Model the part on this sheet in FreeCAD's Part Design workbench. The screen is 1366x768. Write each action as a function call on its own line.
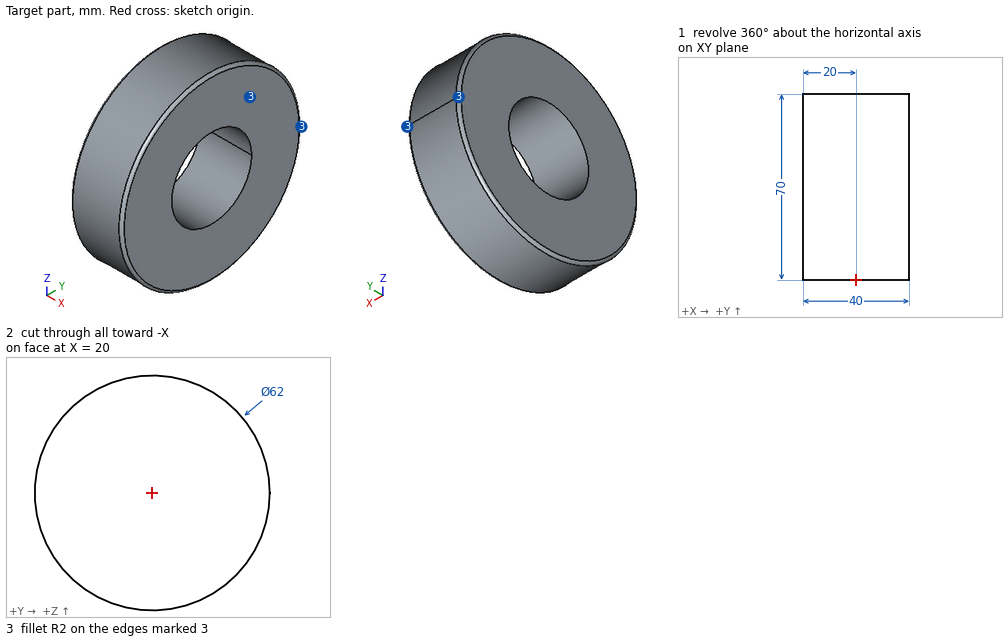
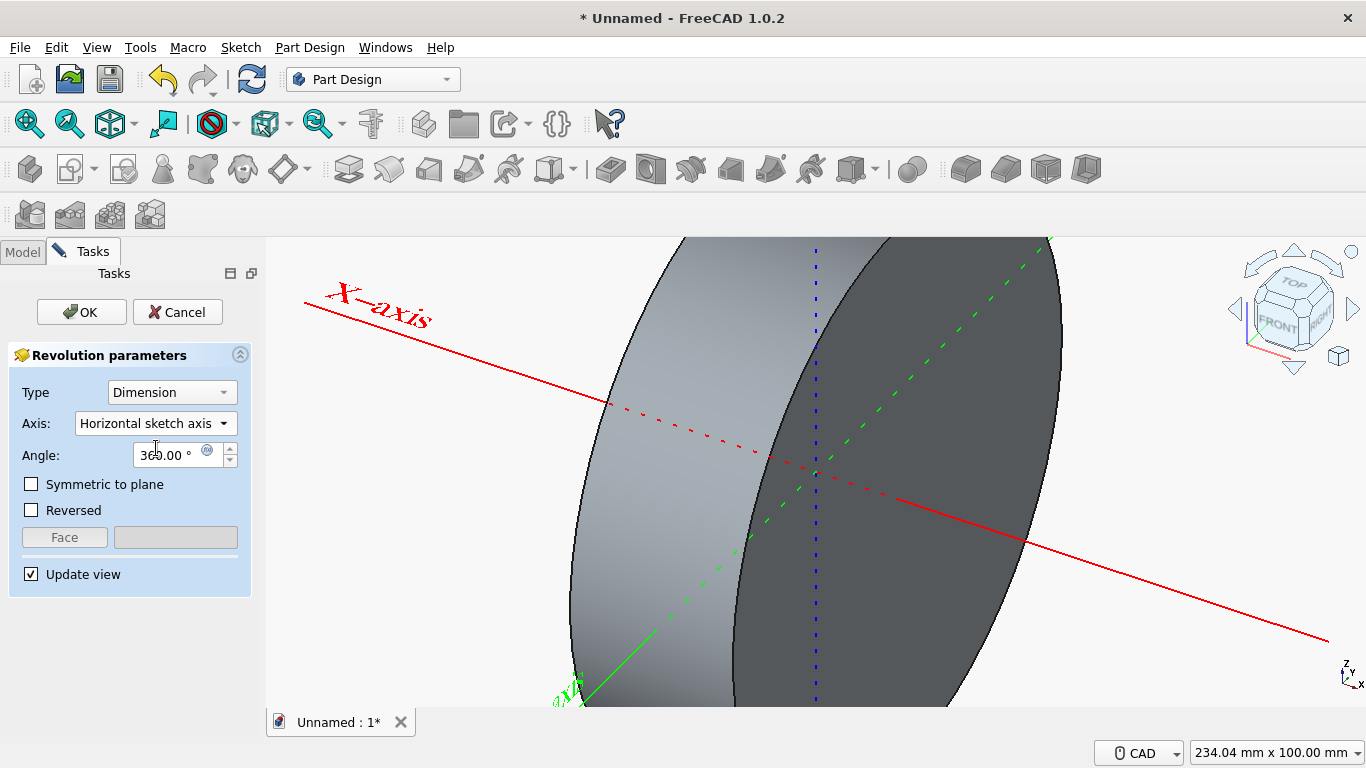
click(82, 312)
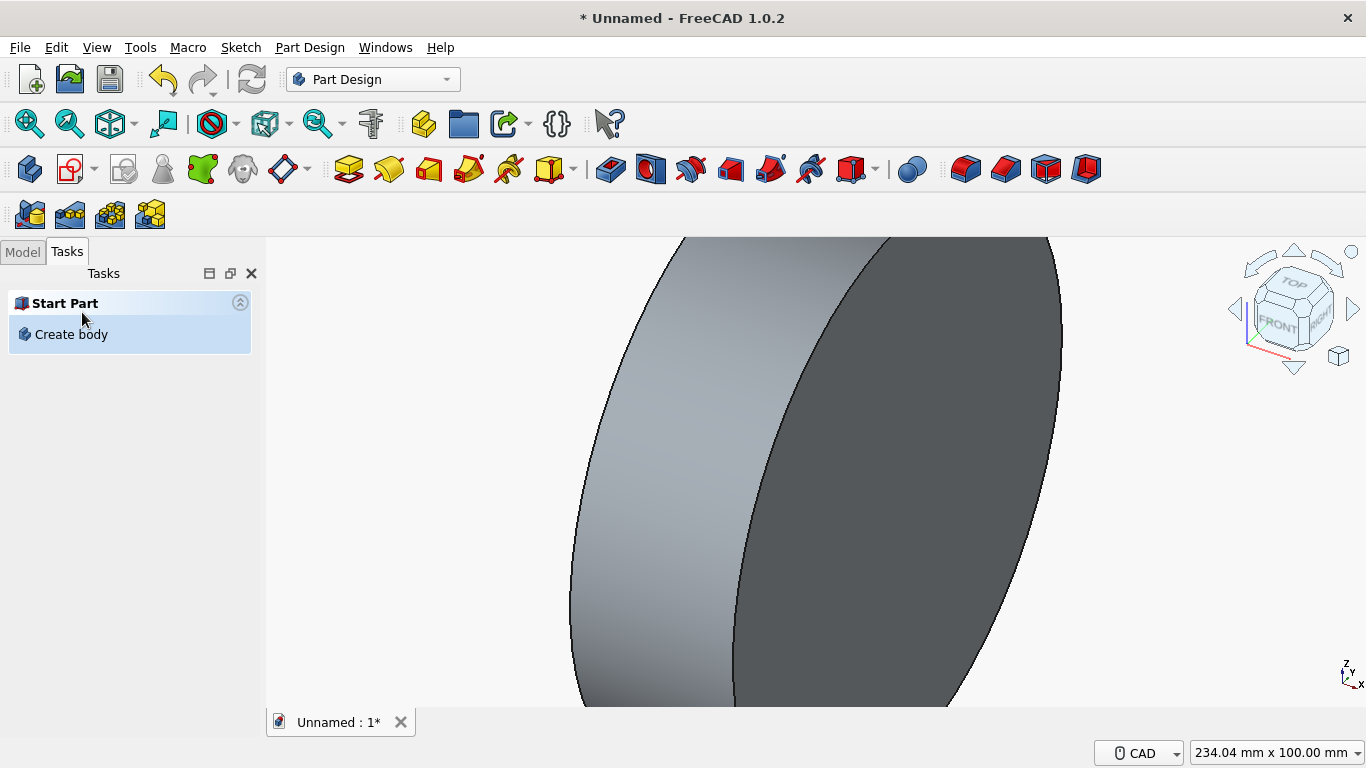
key(v)
key(f)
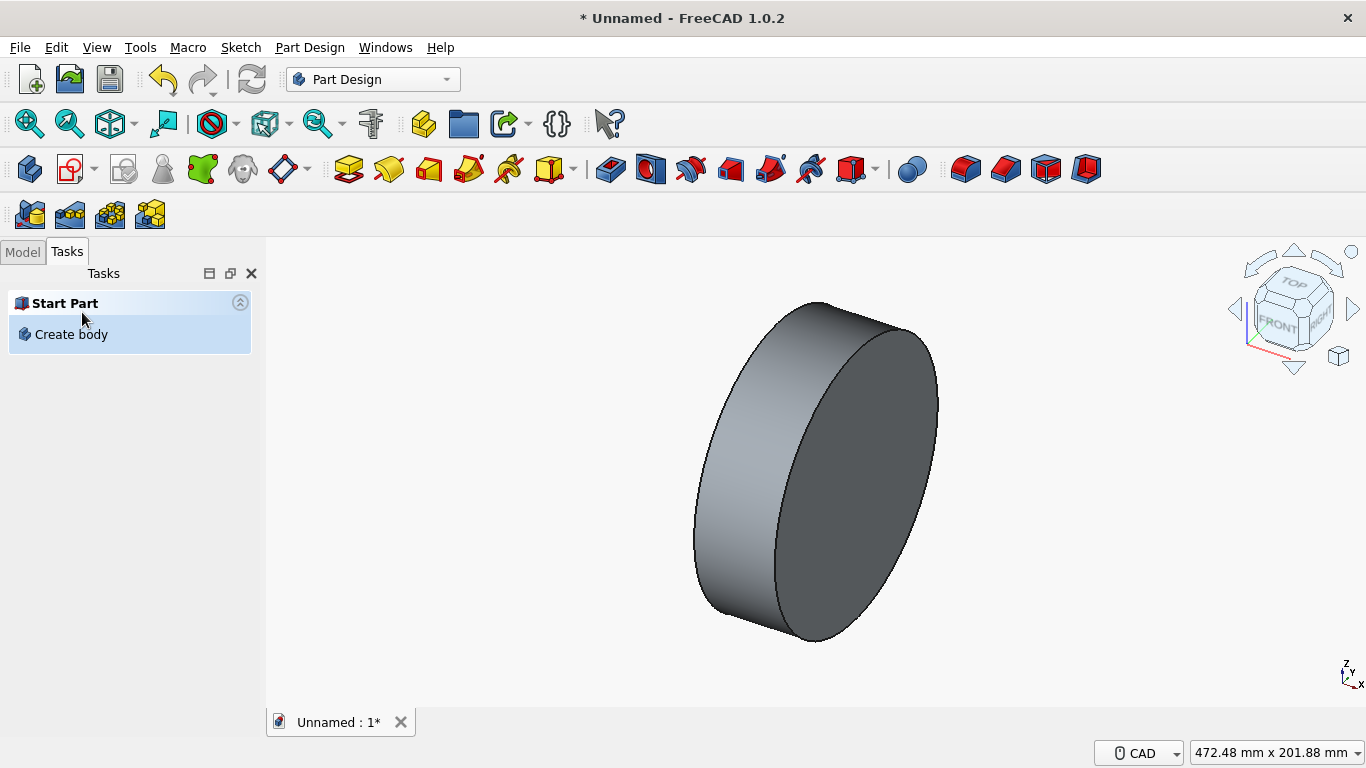
click(856, 484)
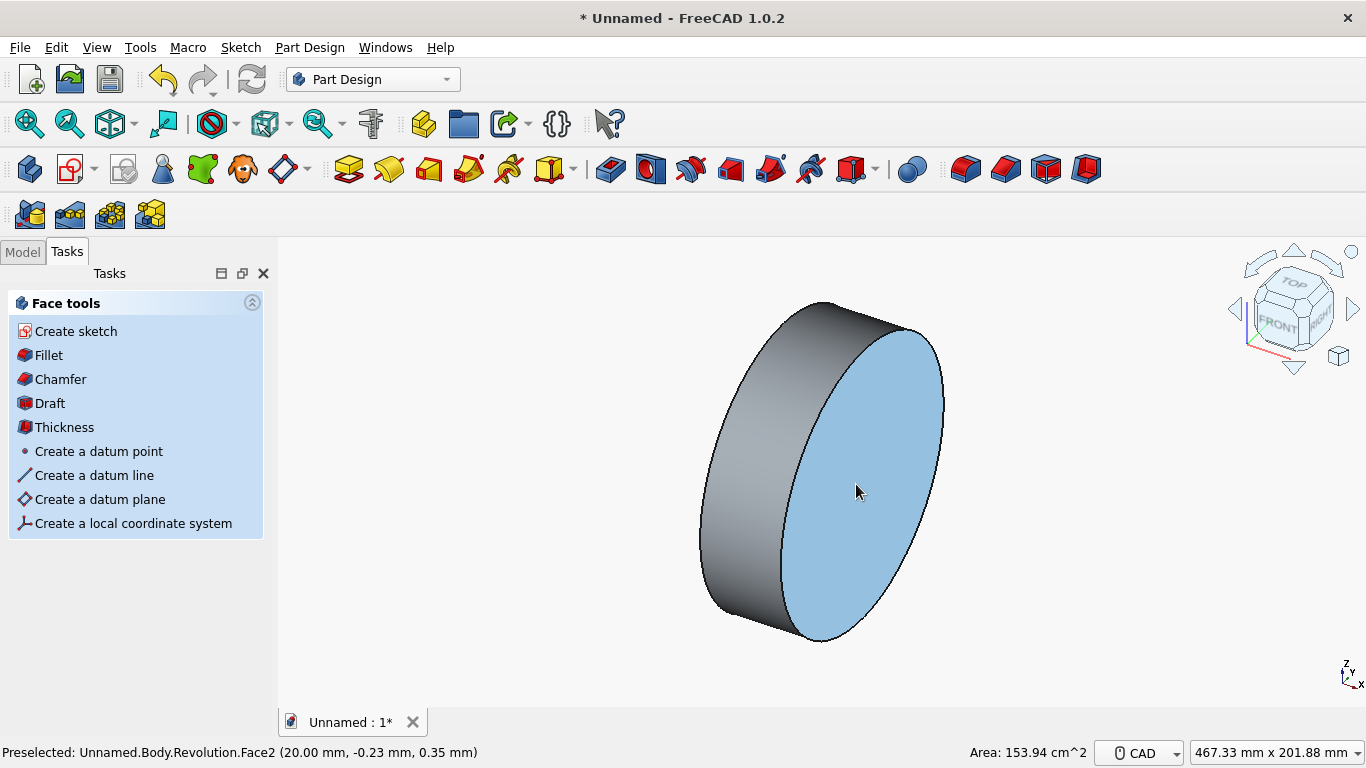
click(70, 170)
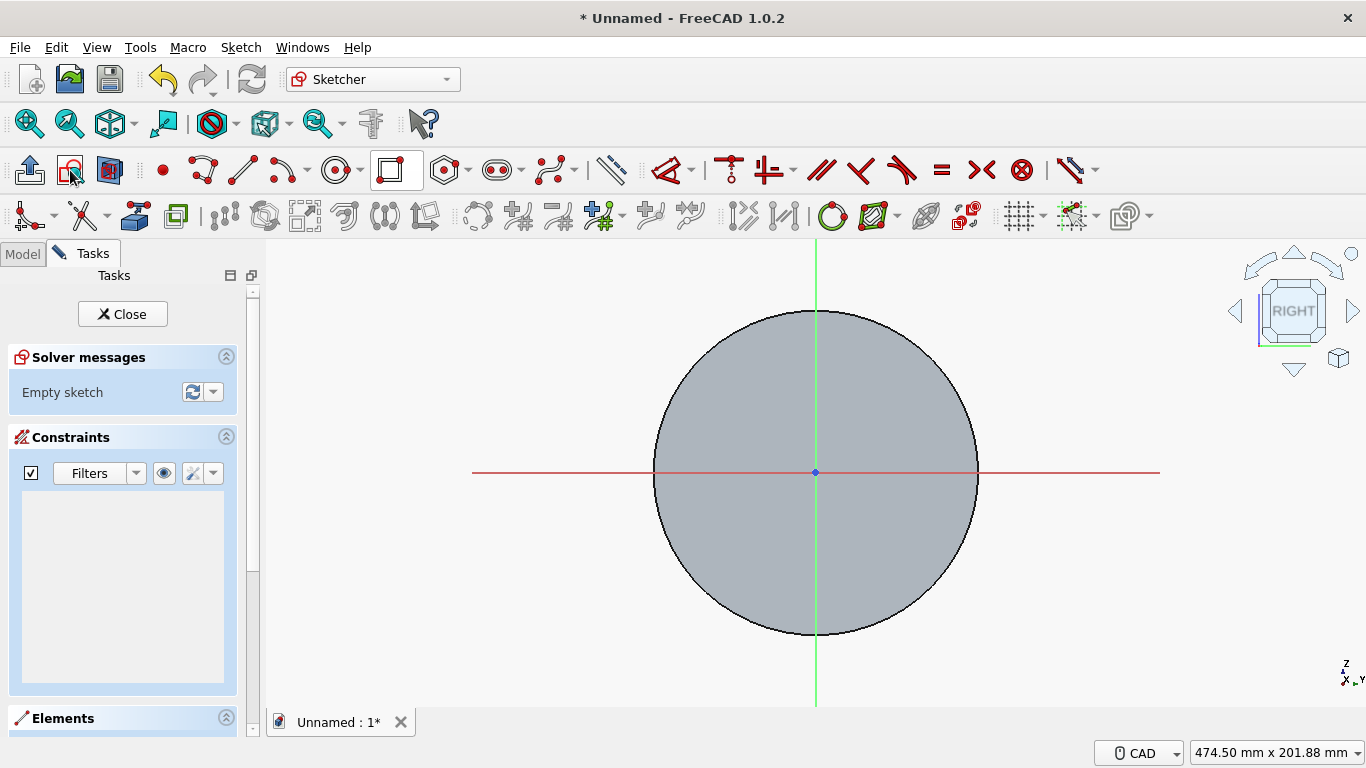
scroll(872, 473, up, 4)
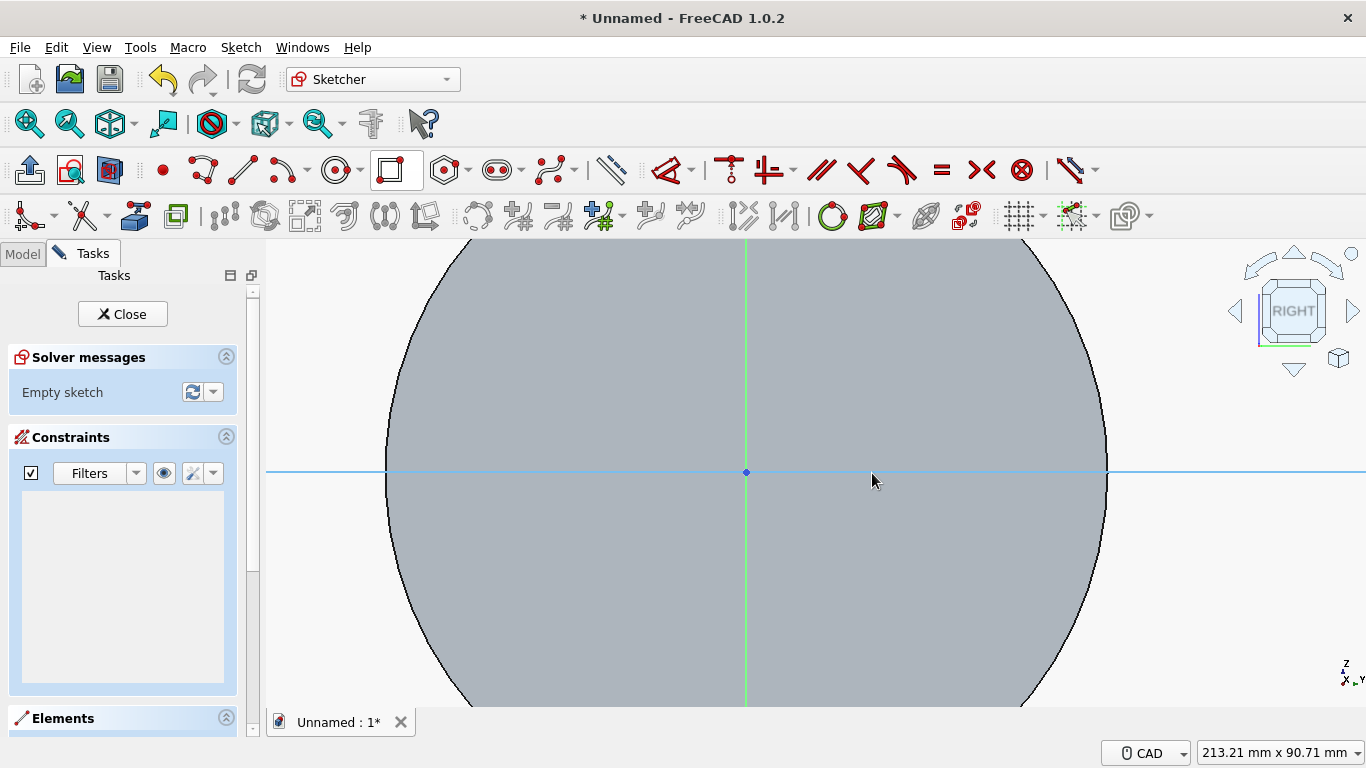
key(g)
key(c)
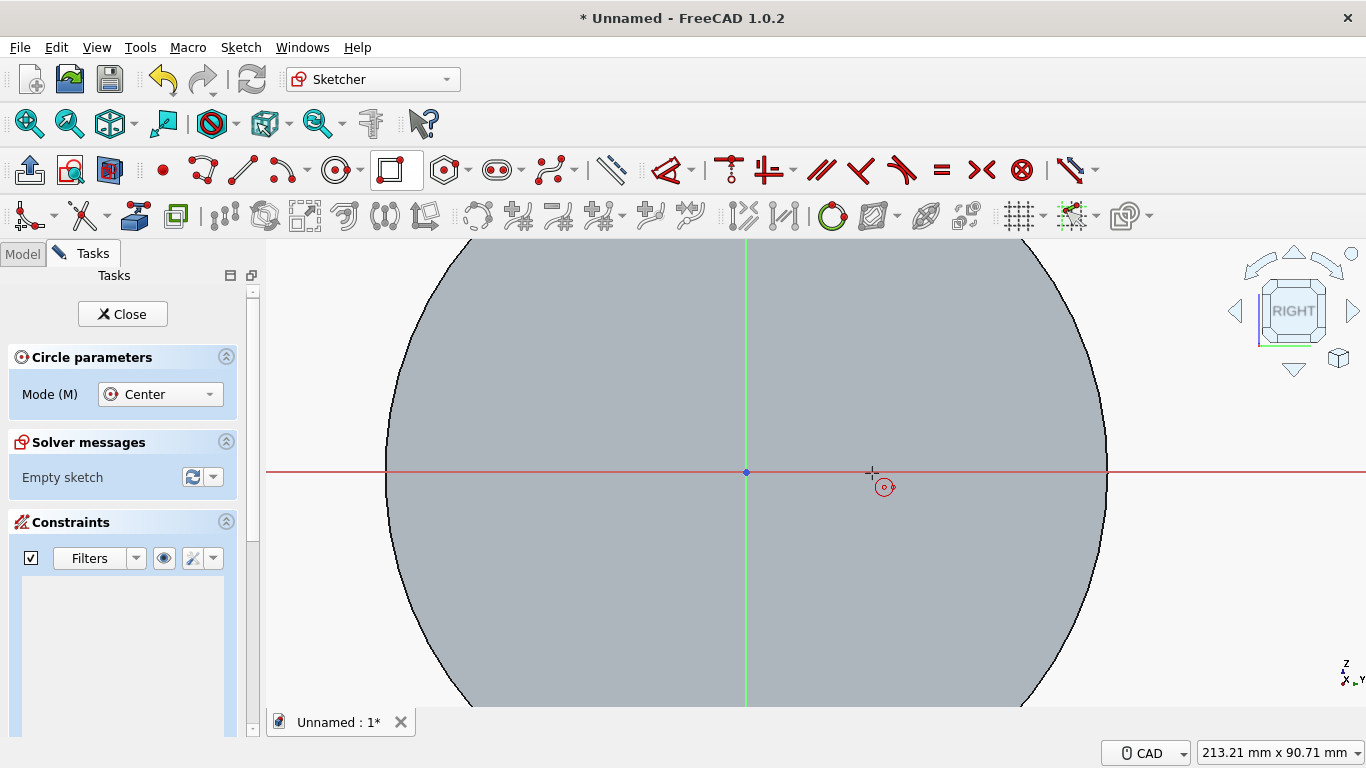
click(746, 472)
move(860, 359)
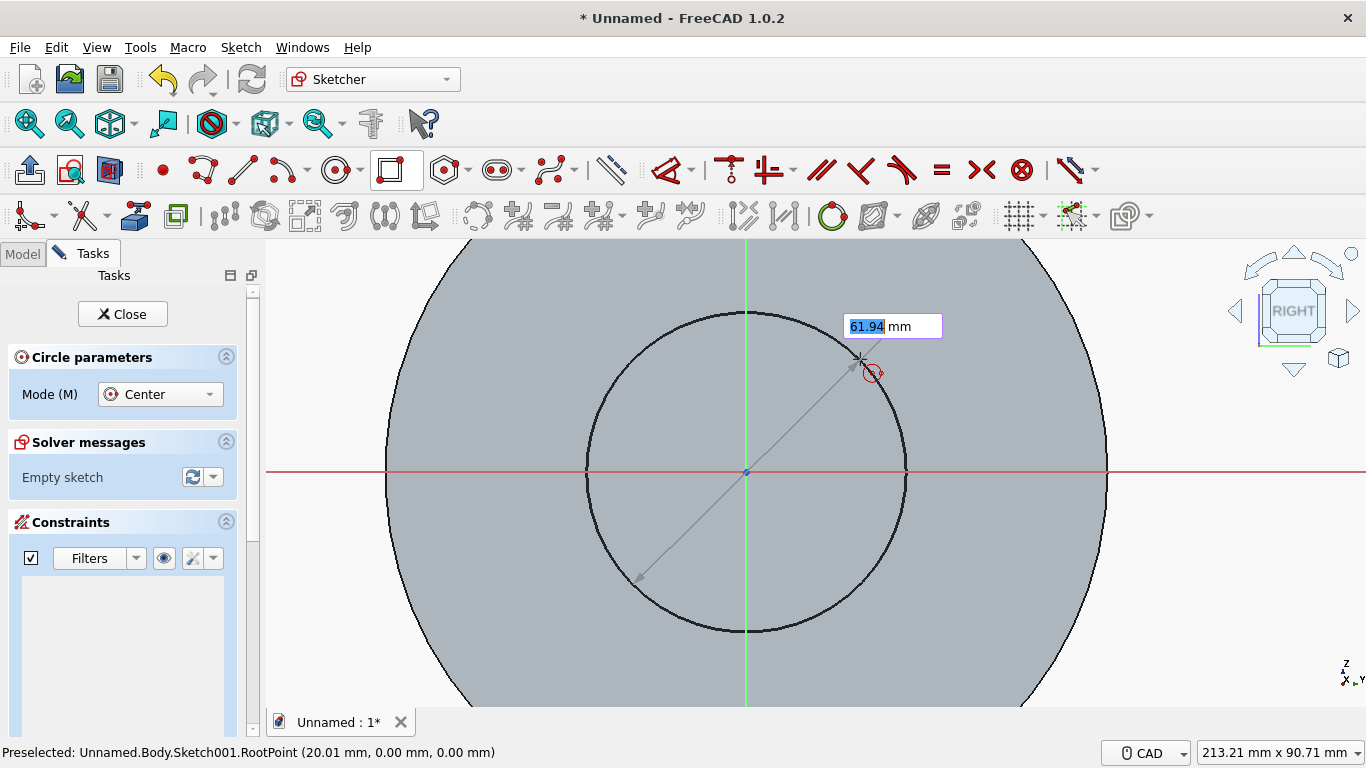
text(62)
key(Return)
key(Escape)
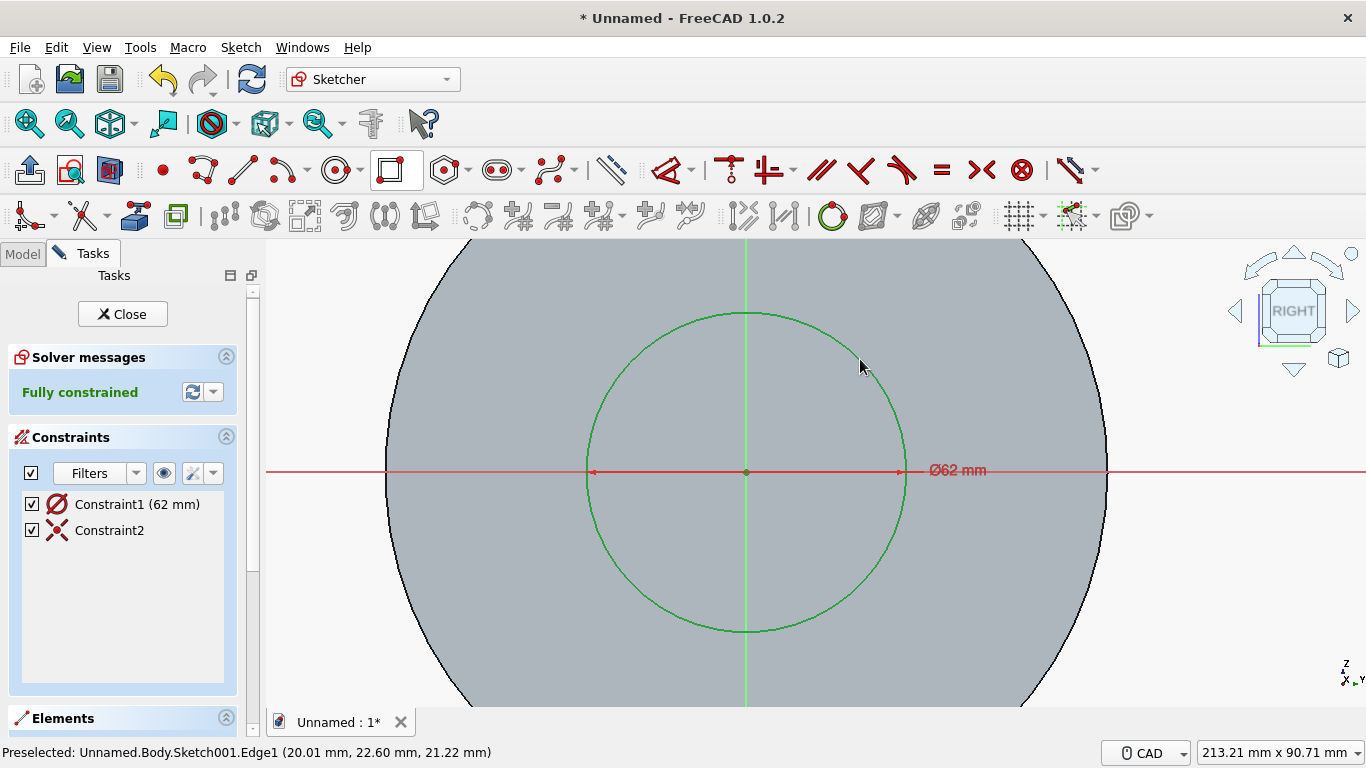
click(123, 314)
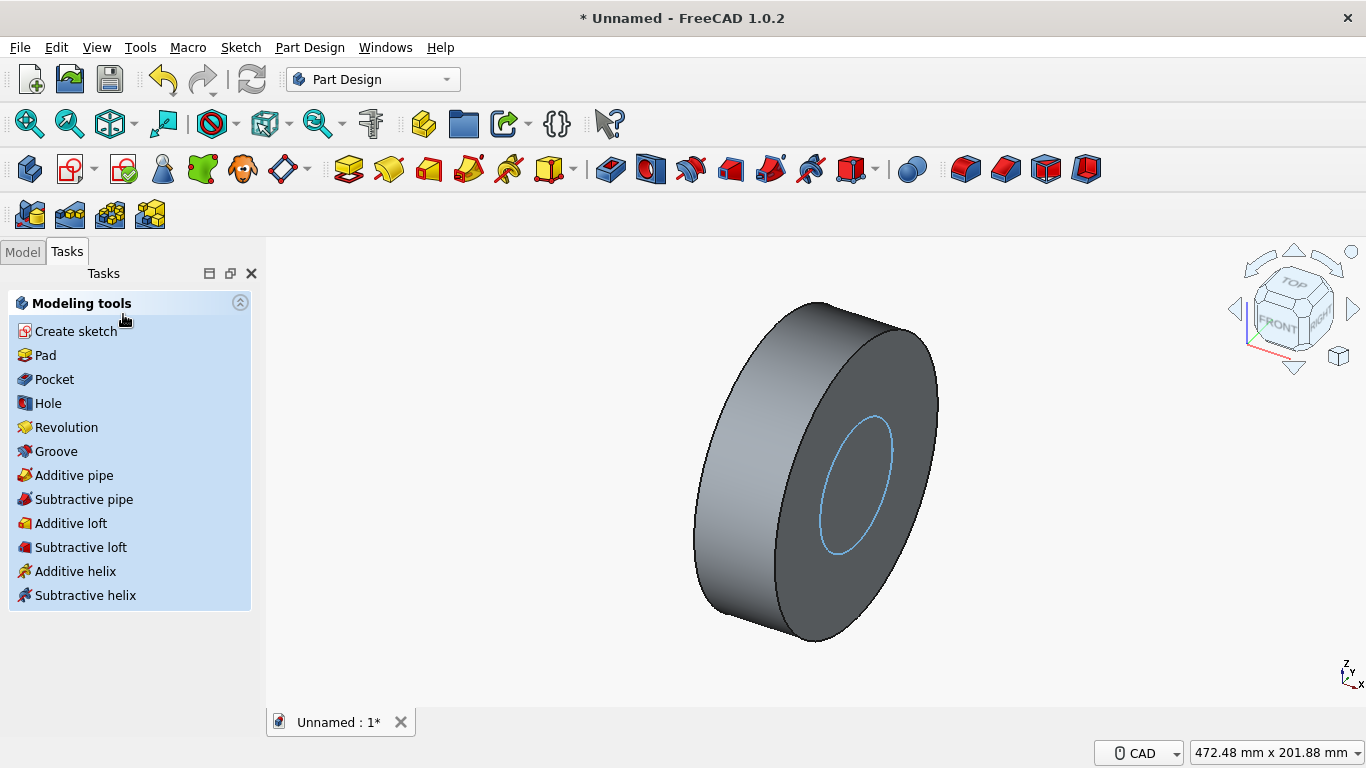
click(612, 170)